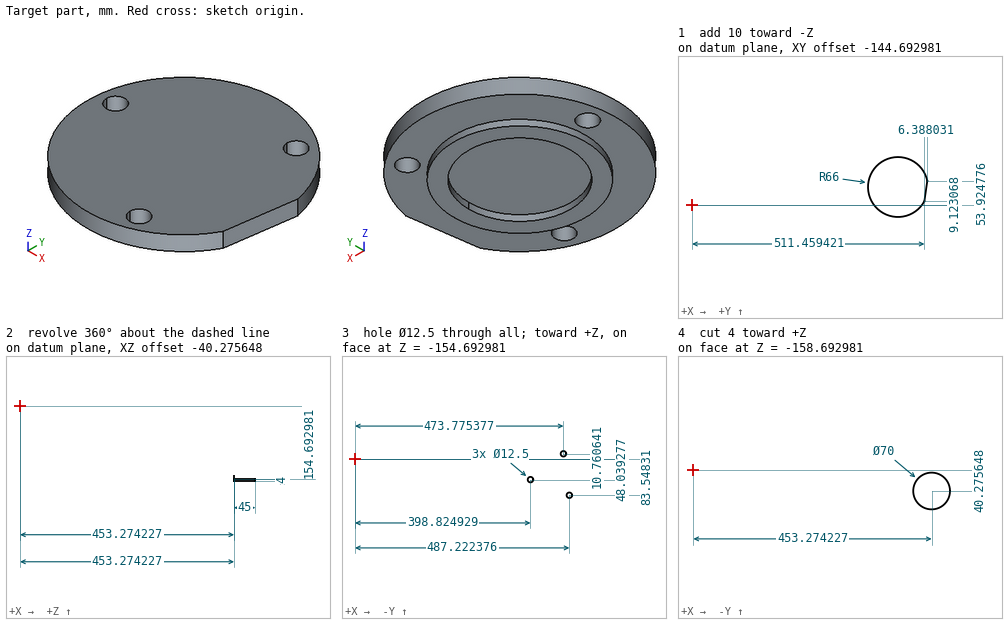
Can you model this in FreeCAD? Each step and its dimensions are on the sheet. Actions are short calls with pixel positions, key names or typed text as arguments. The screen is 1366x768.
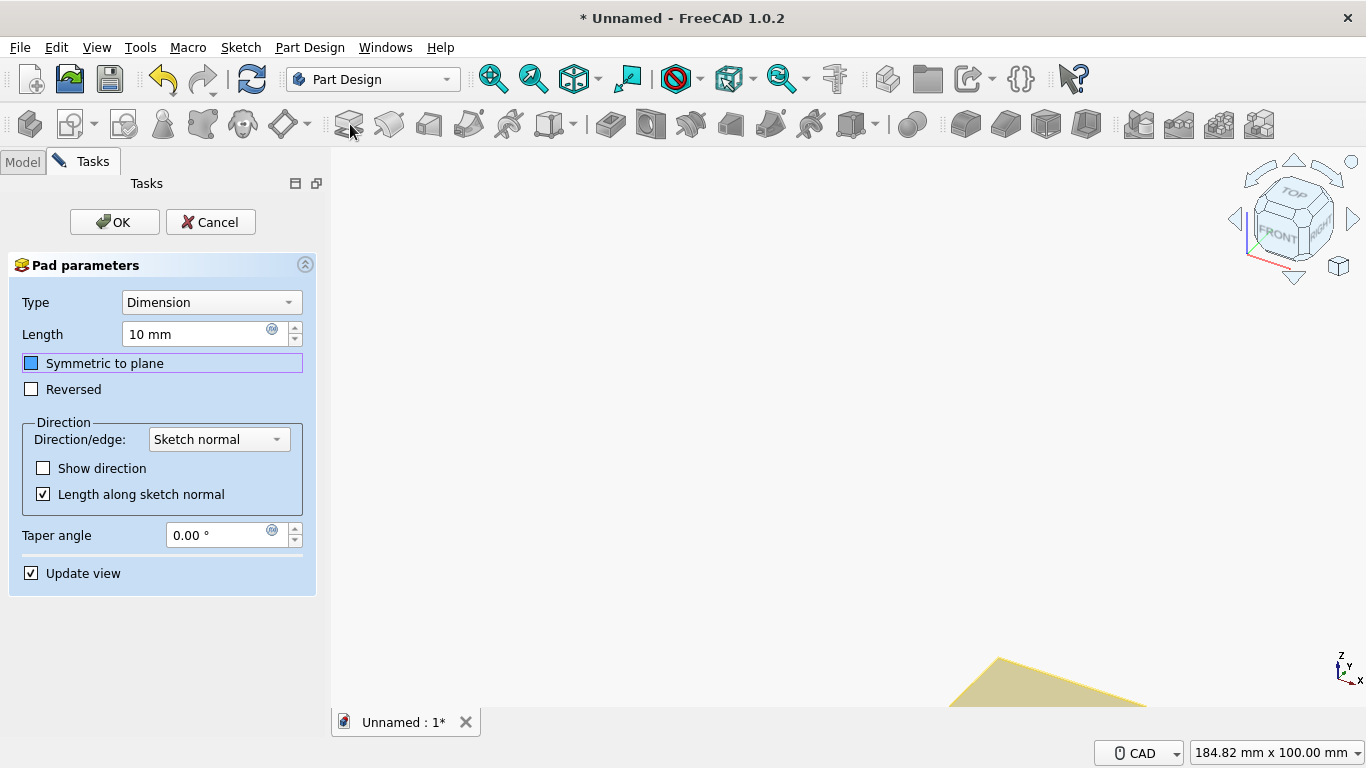
click(30, 389)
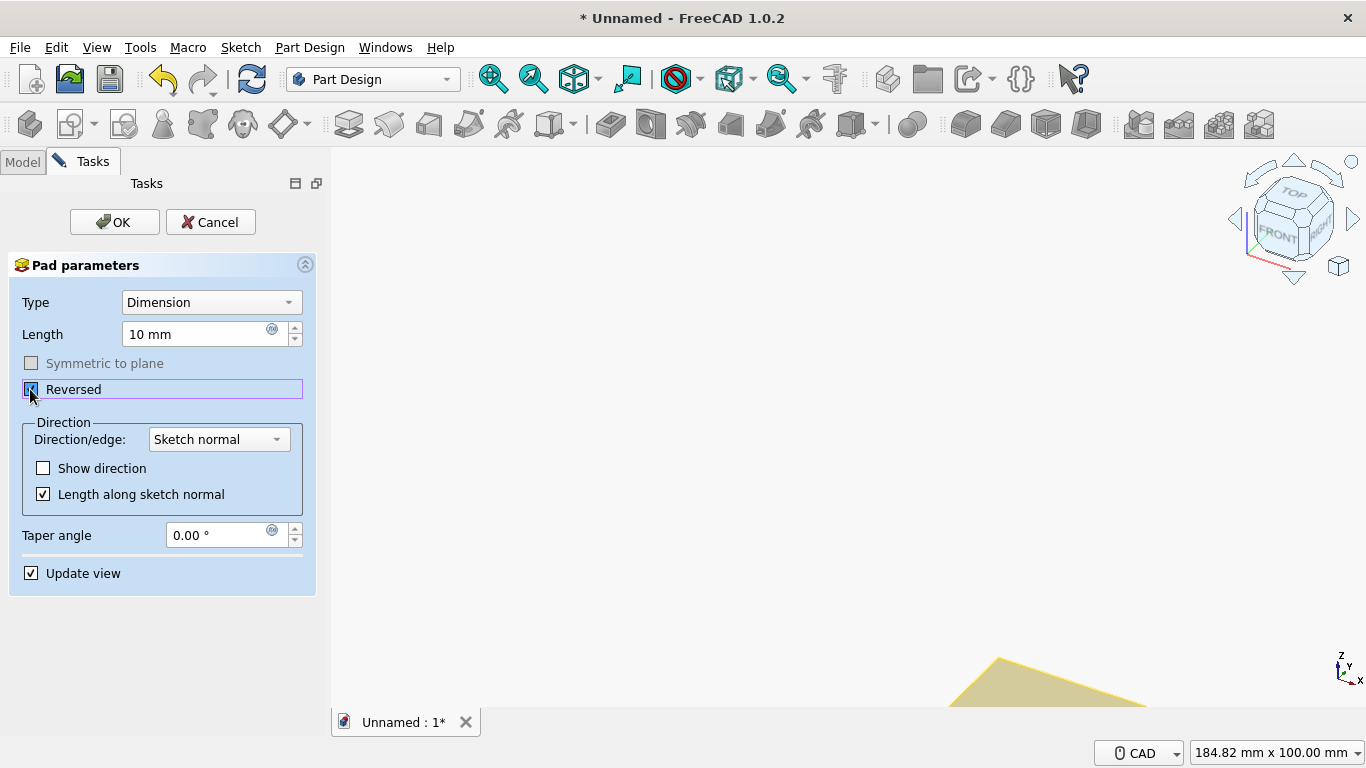
click(115, 222)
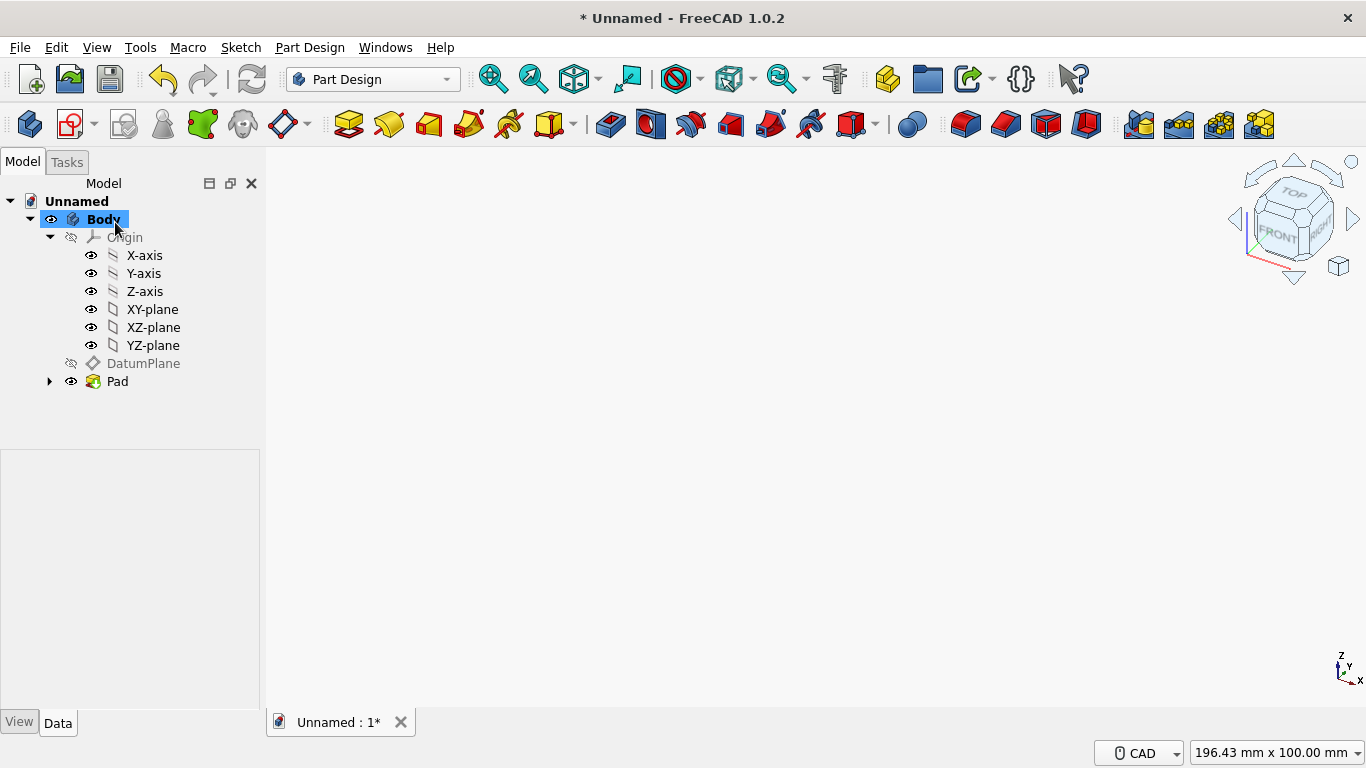
click(494, 80)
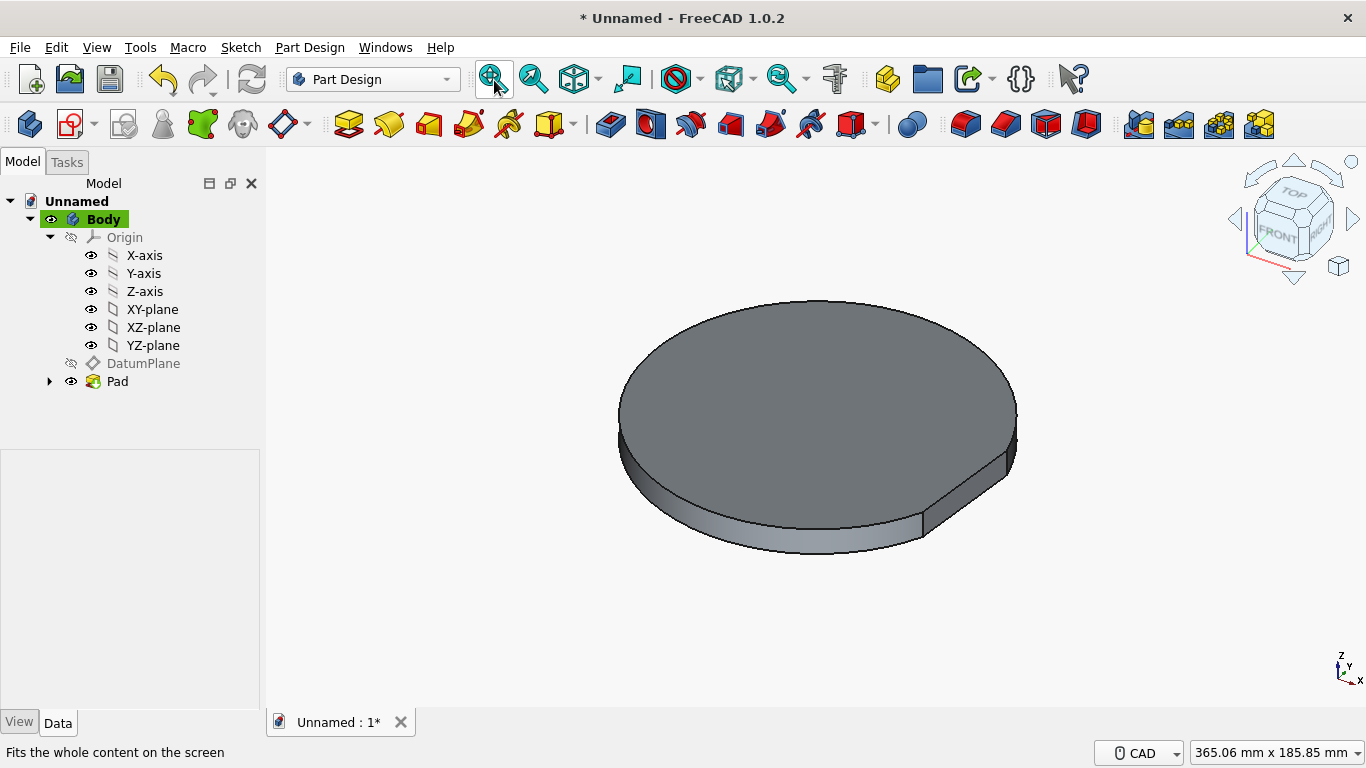
click(136, 327)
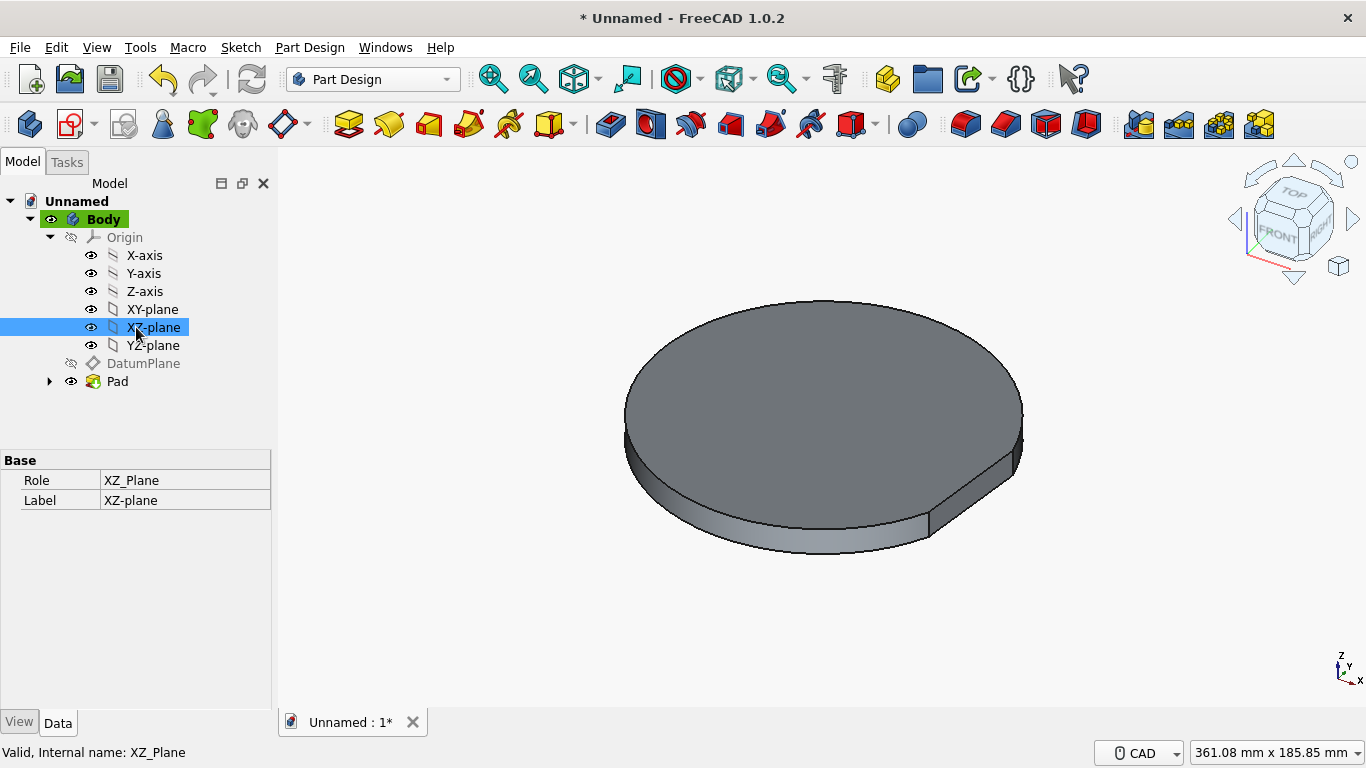
click(284, 124)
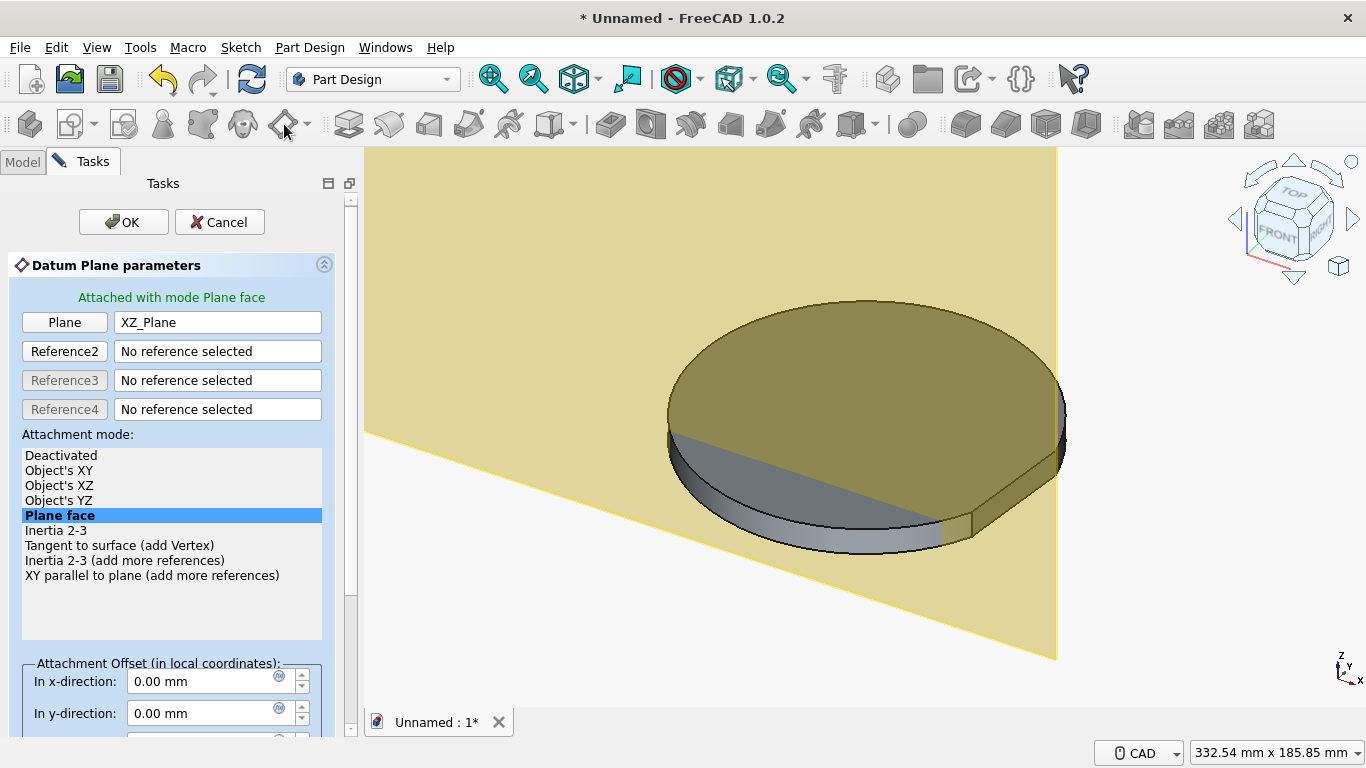
scroll(351, 464, down, 2)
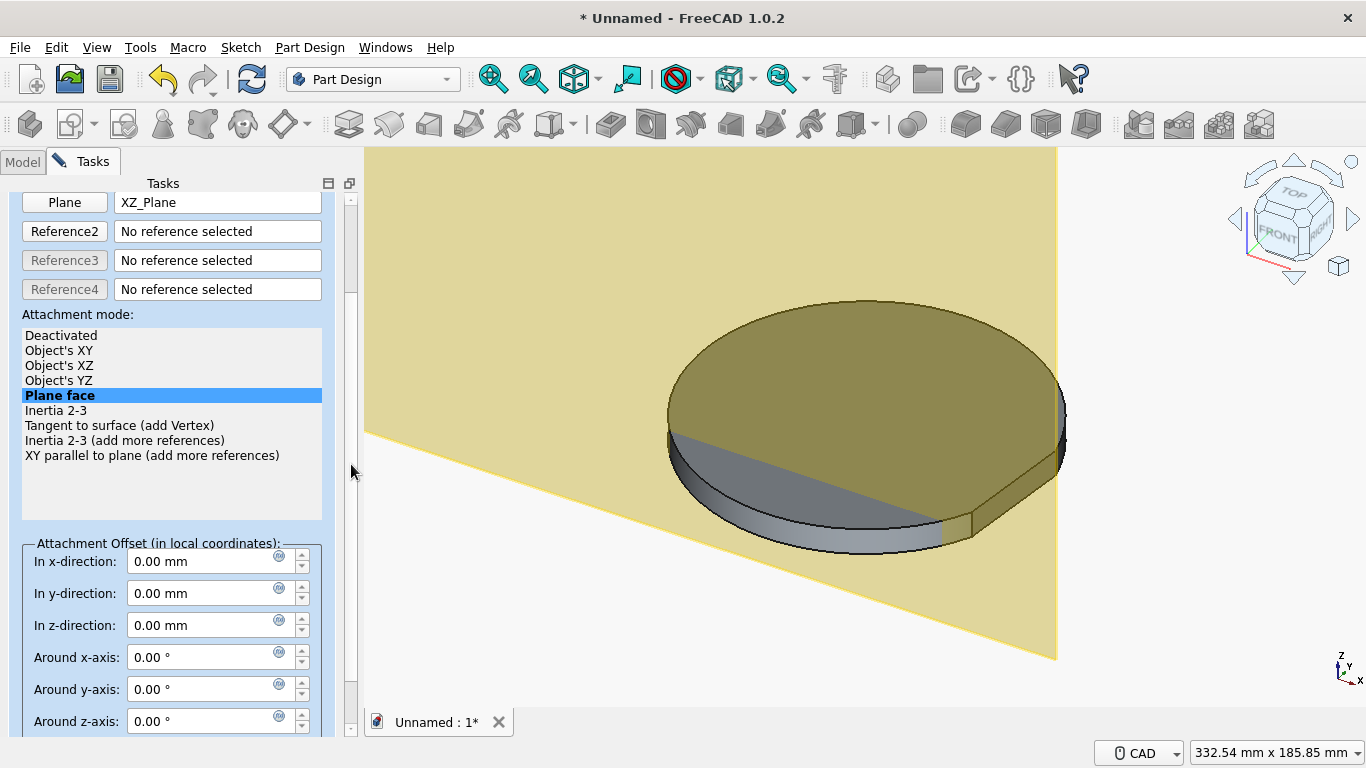
triple_click(210, 625)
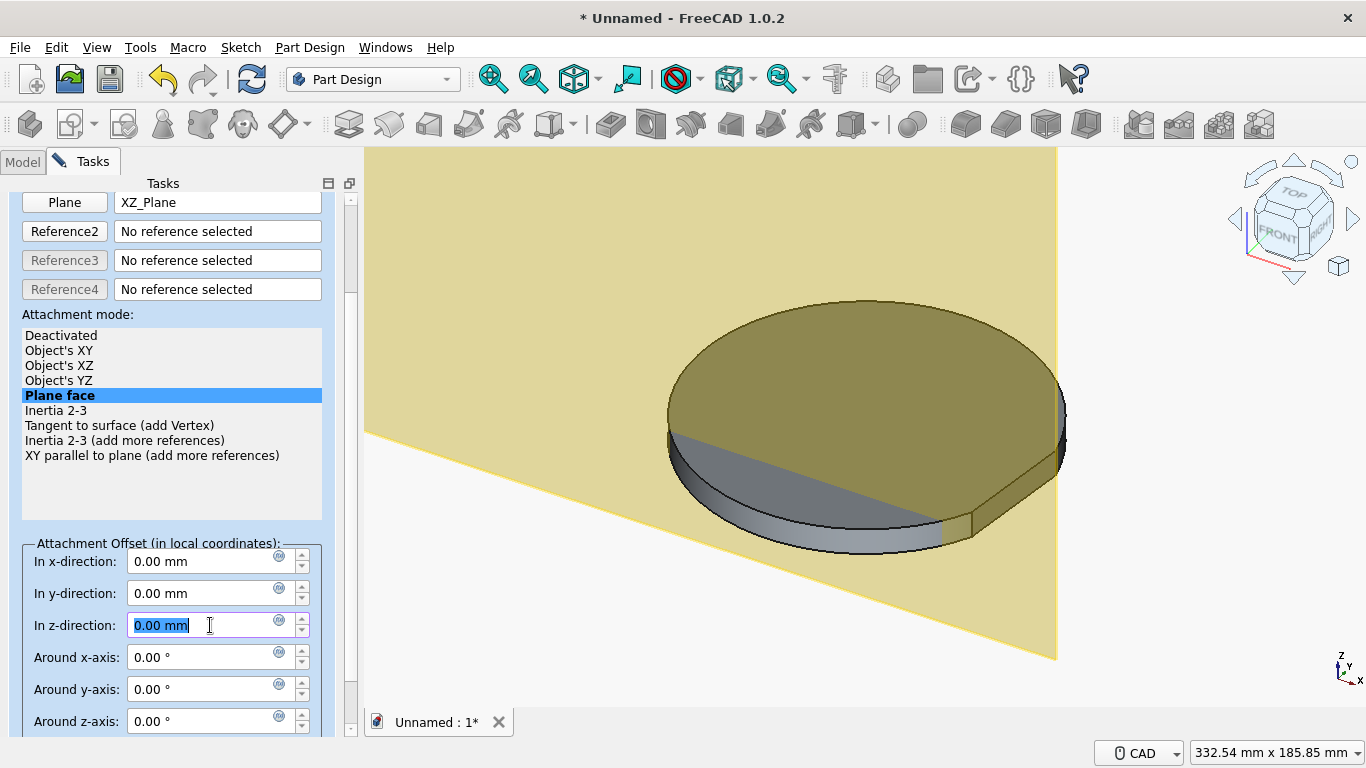
text(-40.275648)
key(Tab)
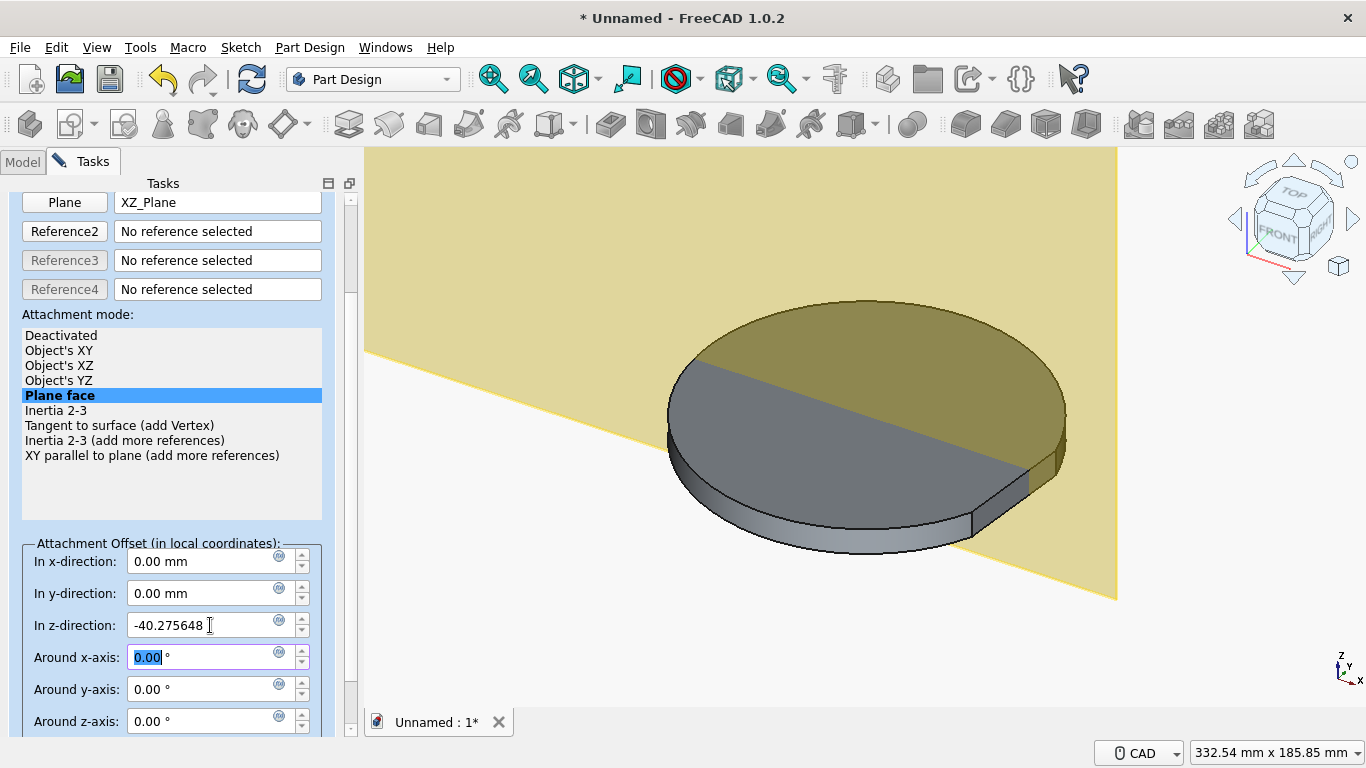
scroll(351, 464, up, 3)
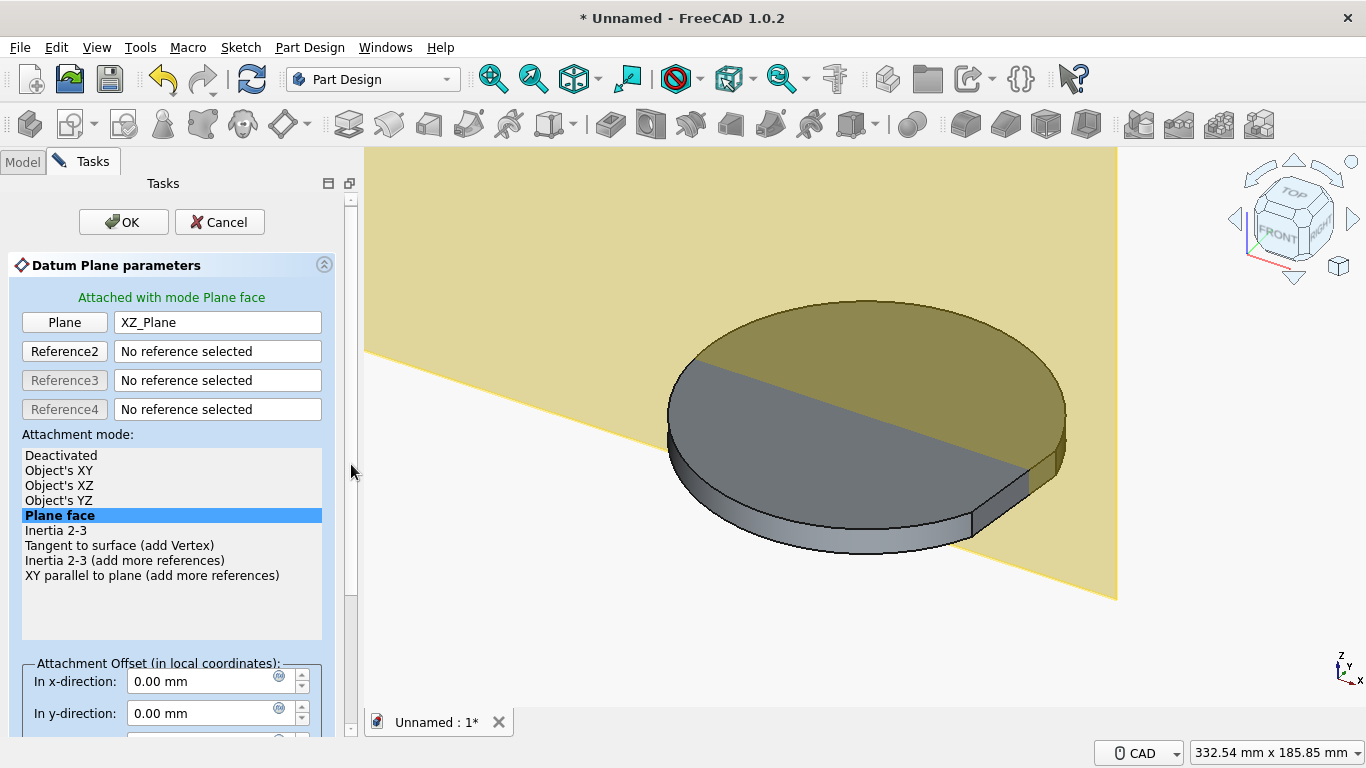
click(124, 222)